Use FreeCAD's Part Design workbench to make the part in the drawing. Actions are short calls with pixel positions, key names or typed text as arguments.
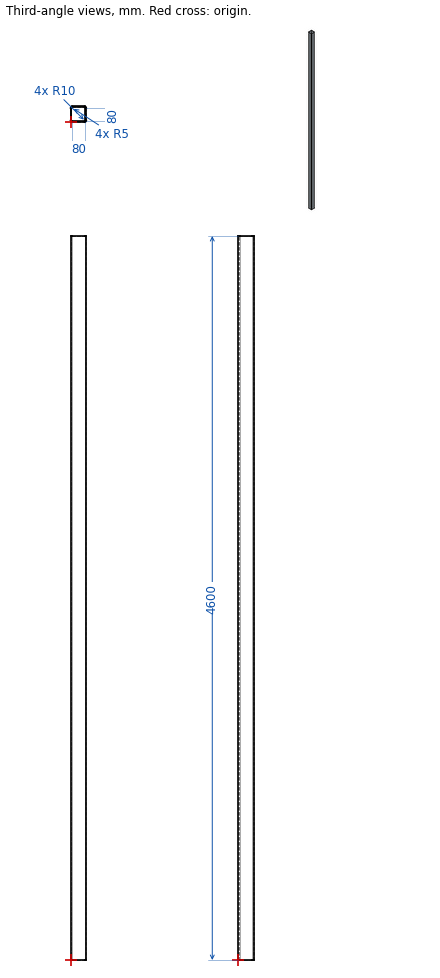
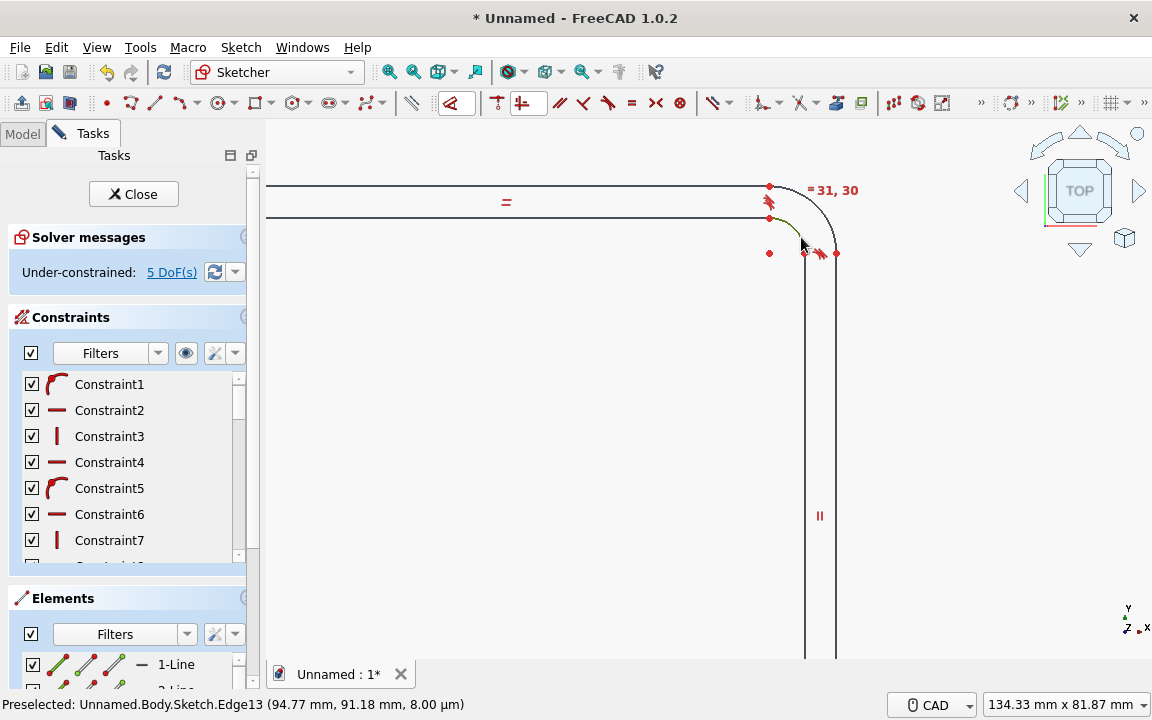
scroll(802, 237, down, 3)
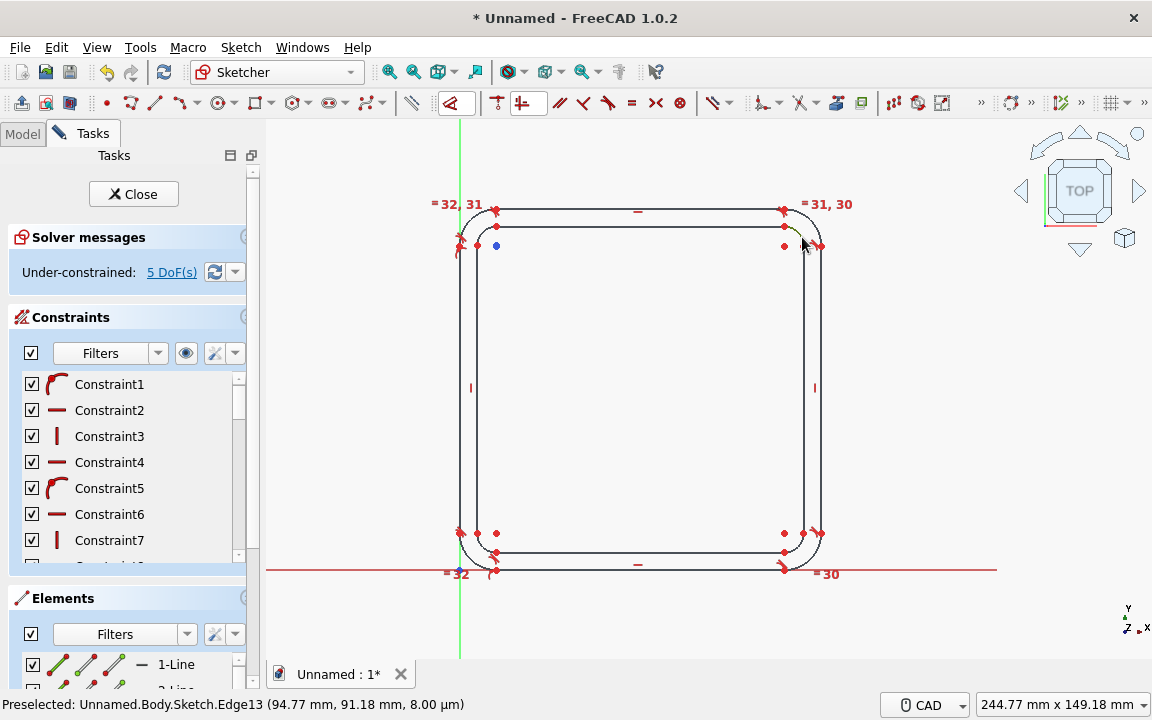
scroll(488, 229, up, 3)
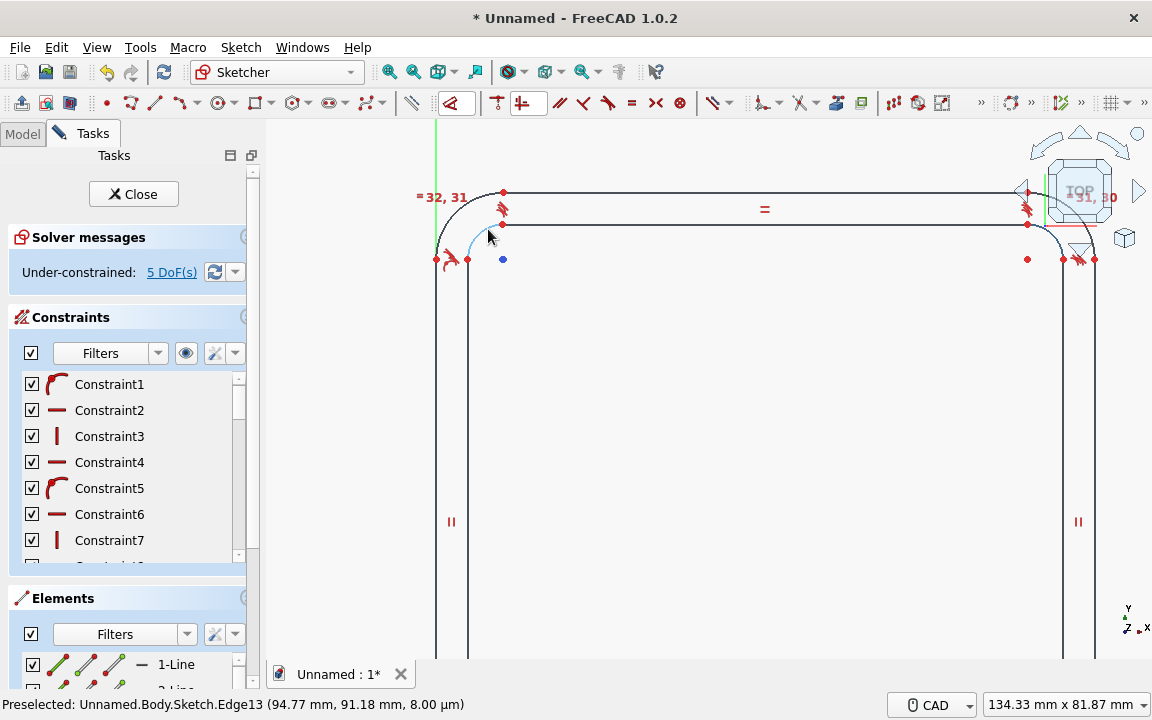
click(487, 228)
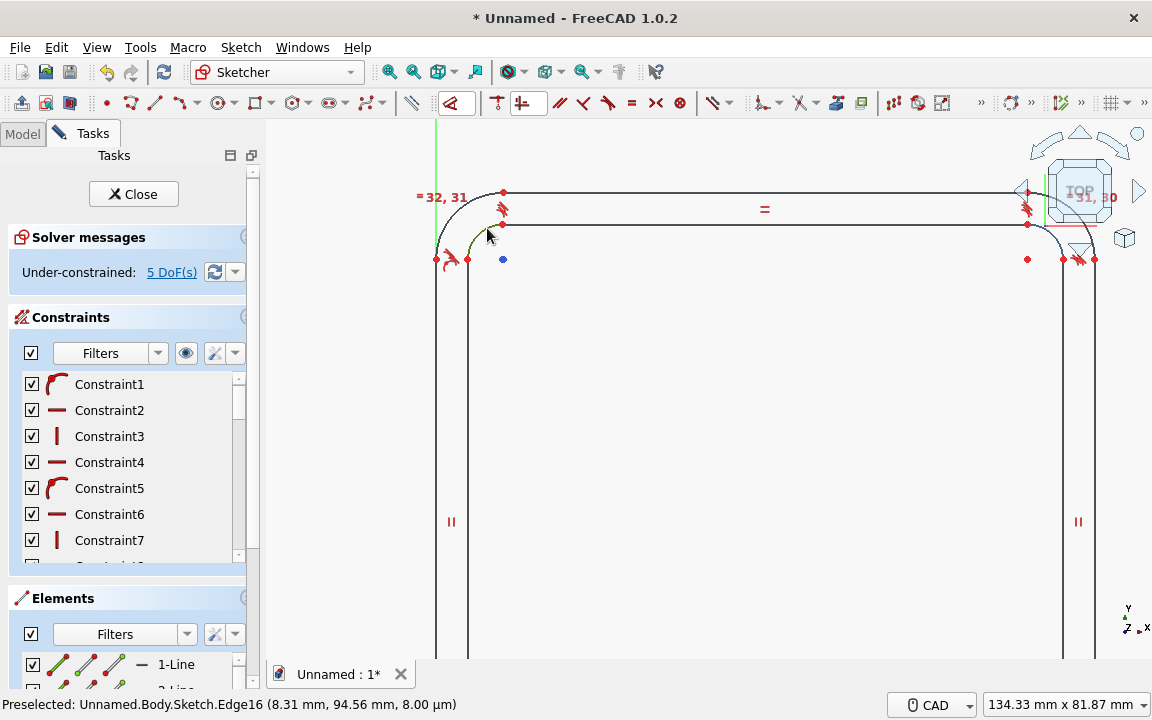
key(e)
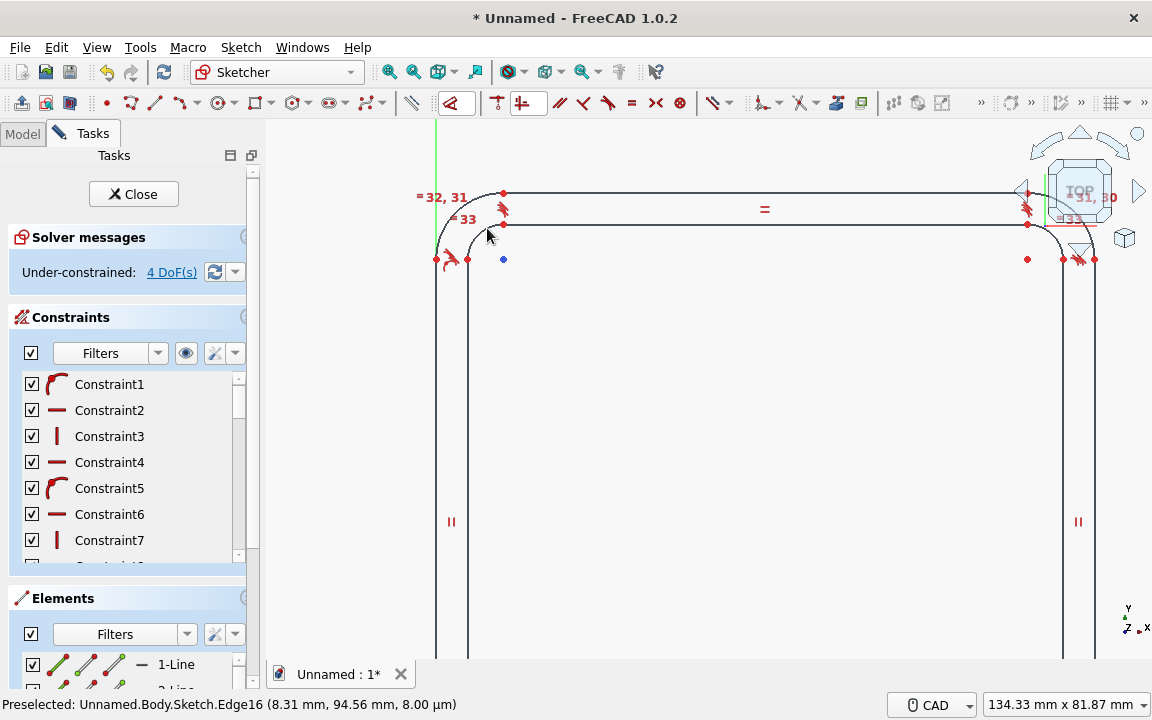
key(d)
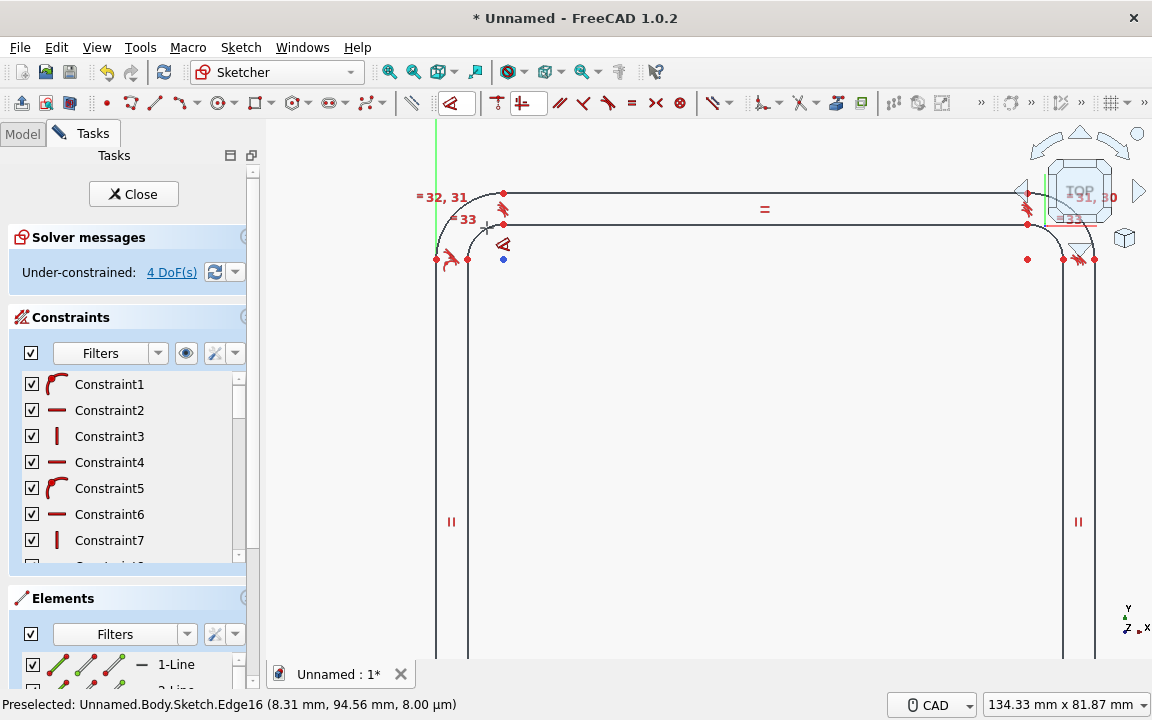
scroll(488, 229, down, 3)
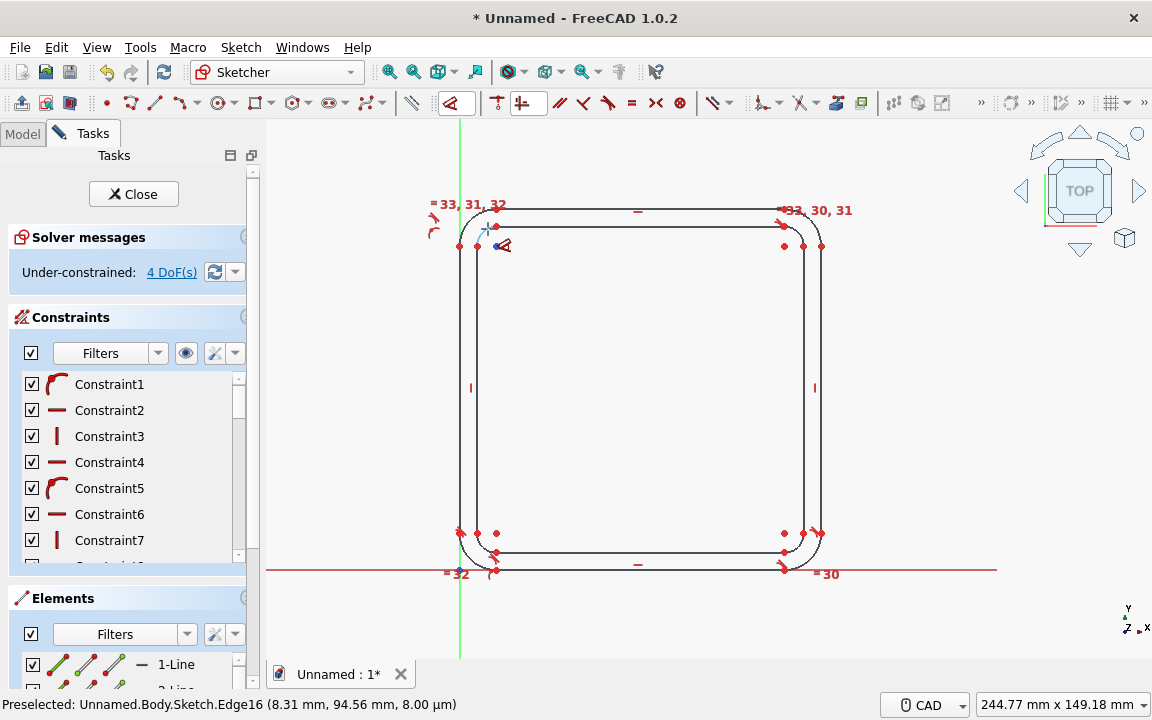
click(817, 550)
click(823, 590)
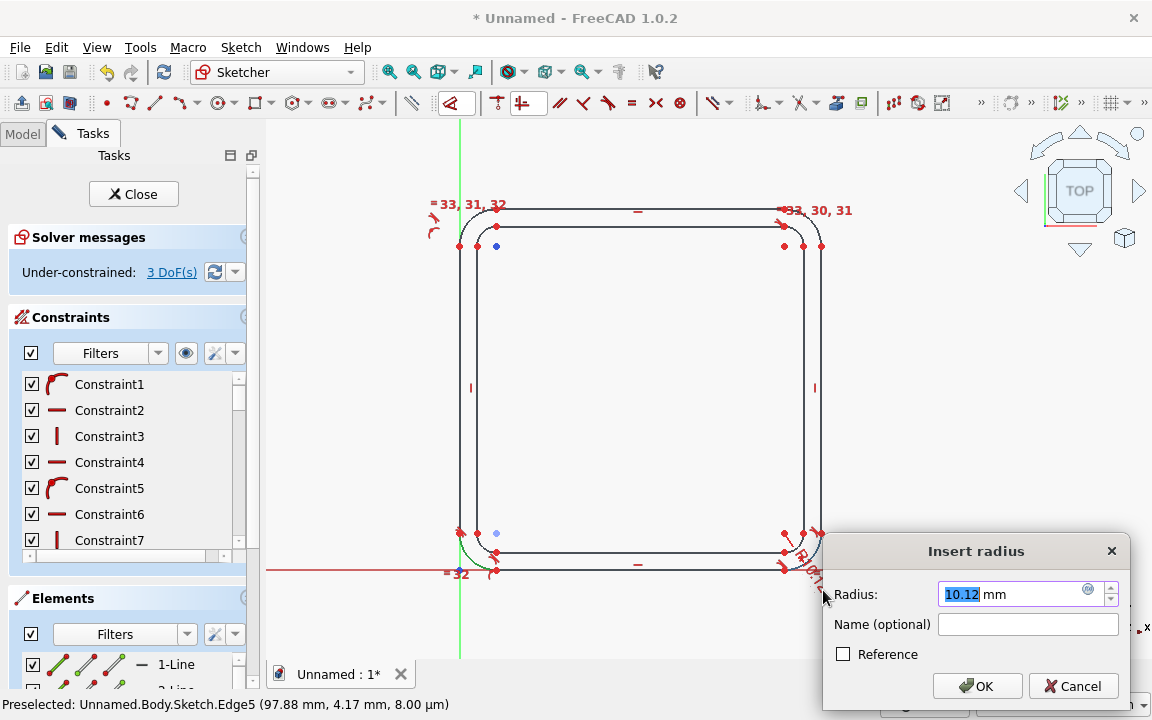
text(10)
key(Return)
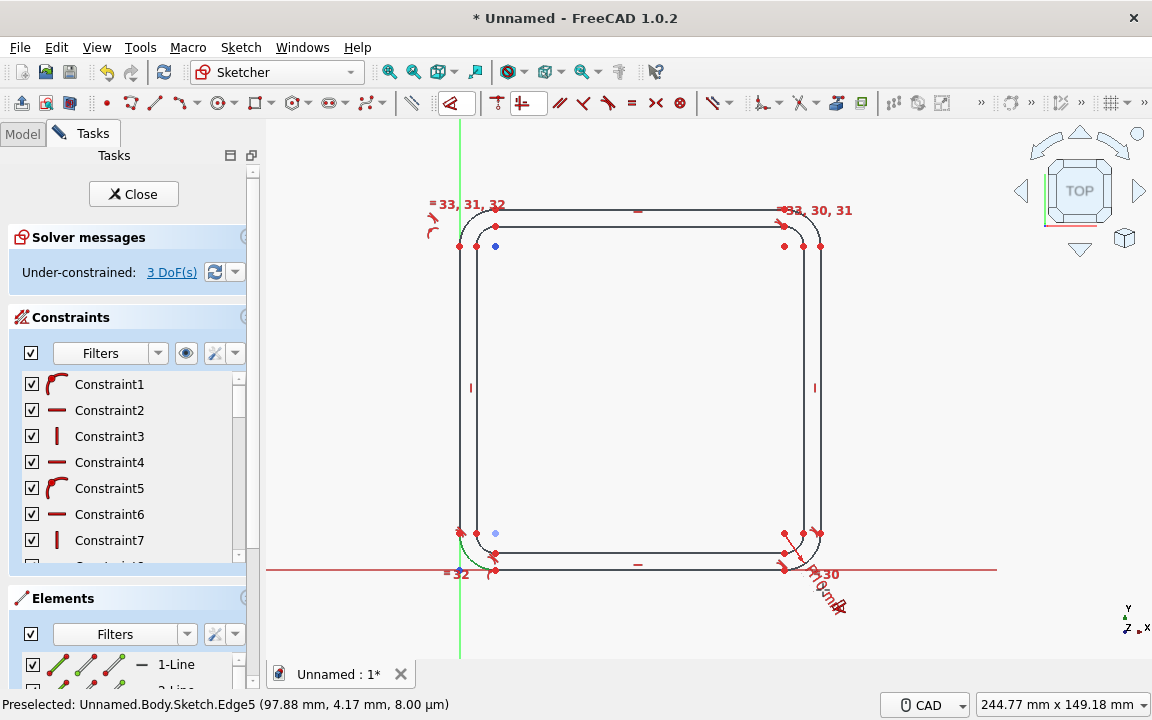
scroll(802, 237, up, 4)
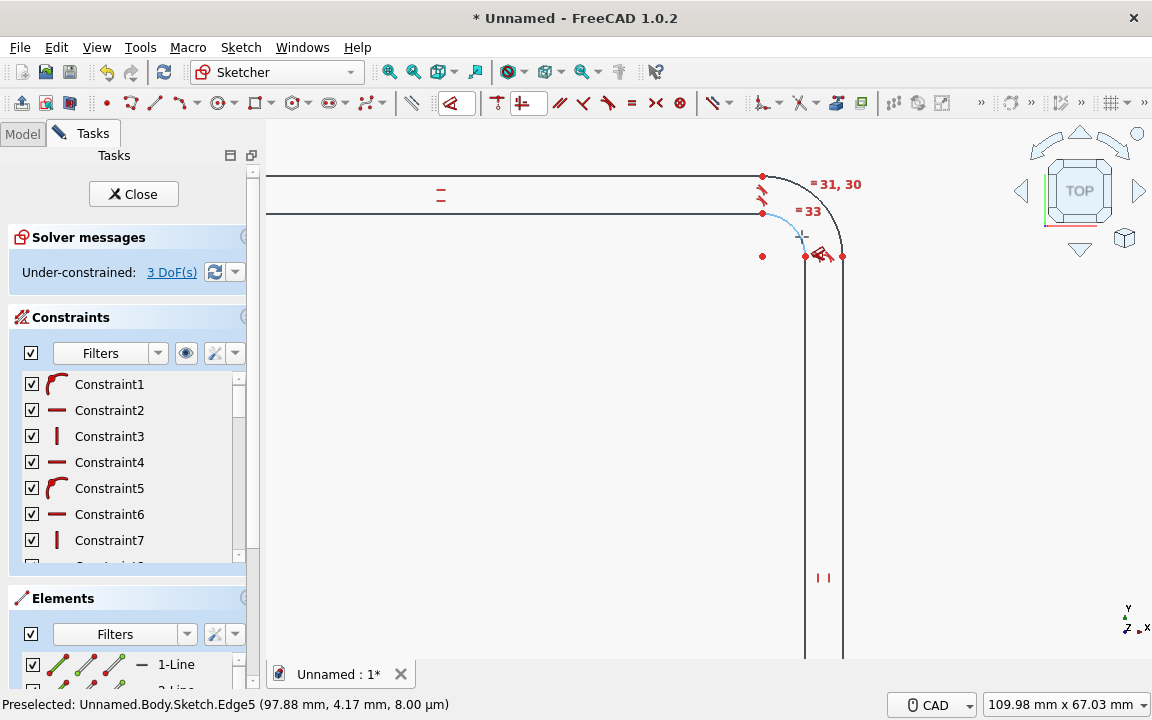
click(800, 237)
click(827, 294)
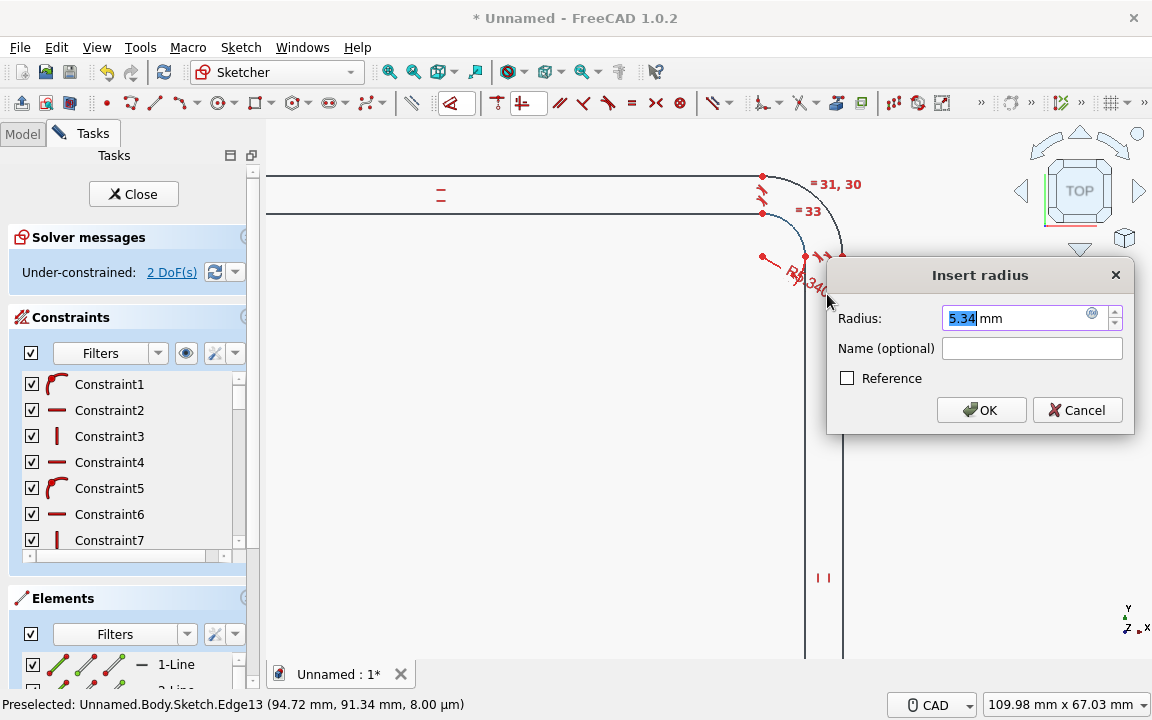
text(5)
key(Return)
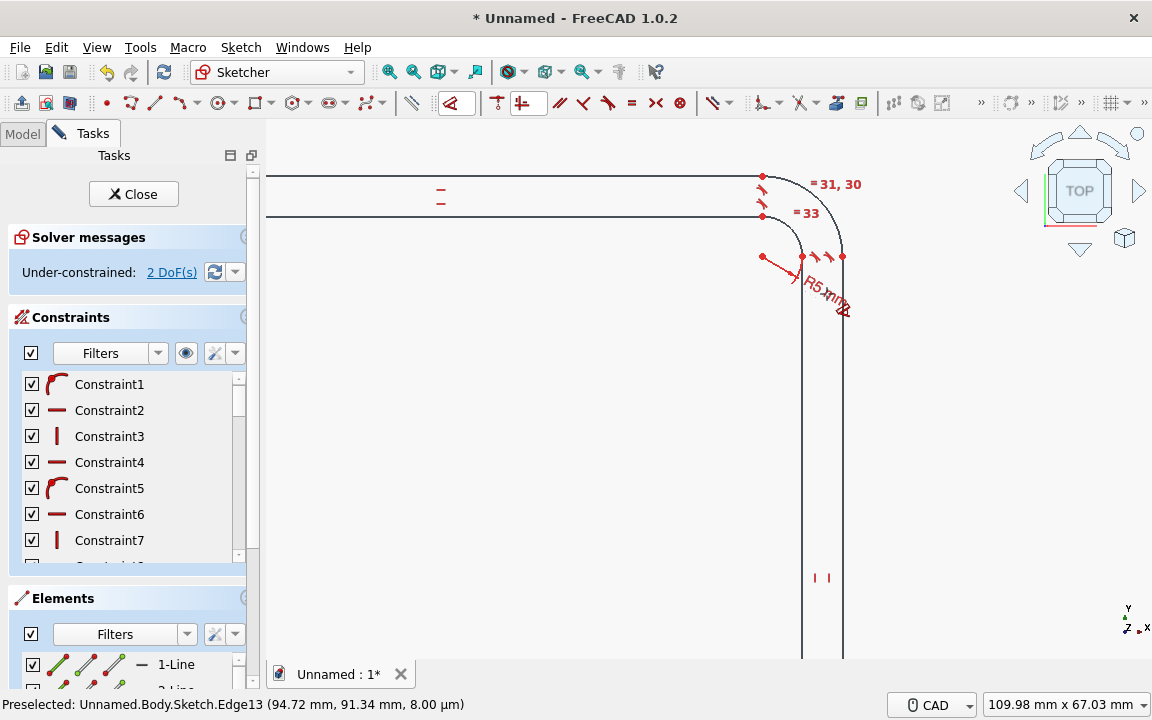
scroll(802, 237, down, 4)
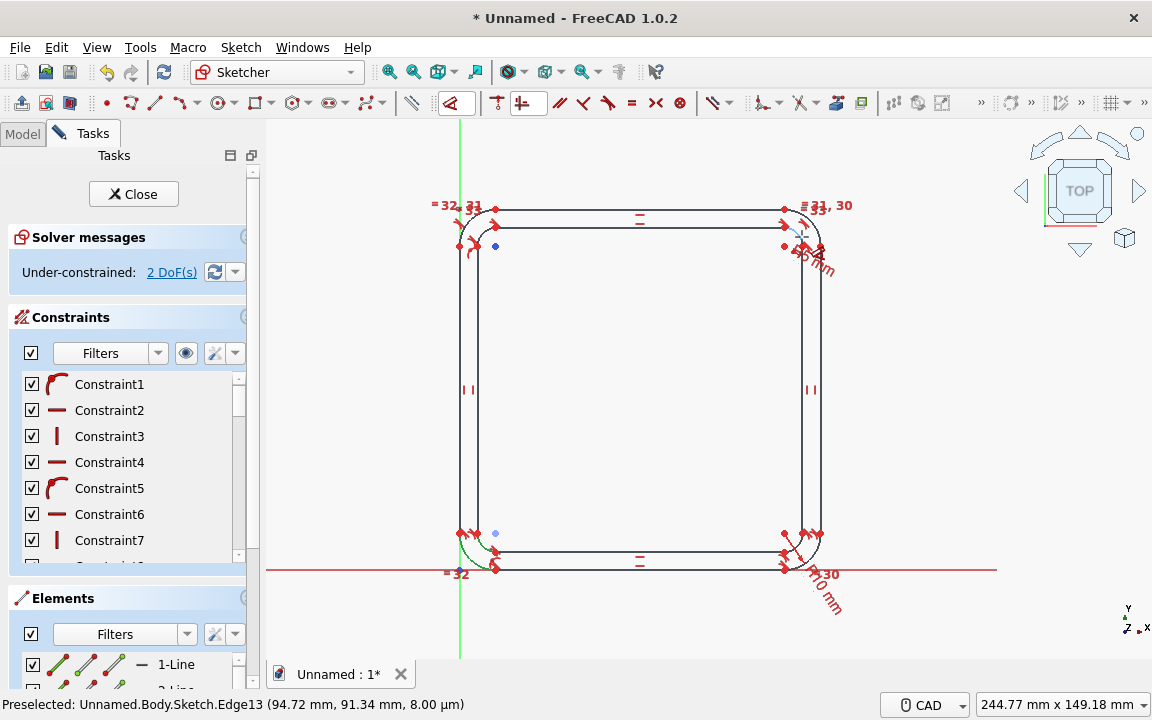
click(582, 570)
click(640, 604)